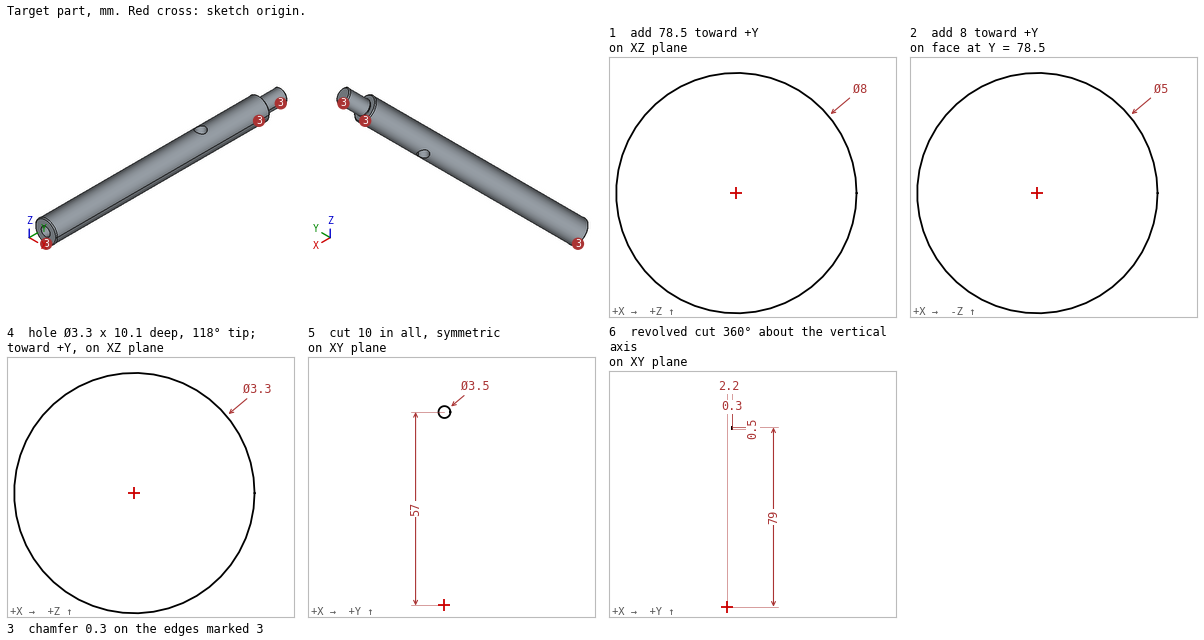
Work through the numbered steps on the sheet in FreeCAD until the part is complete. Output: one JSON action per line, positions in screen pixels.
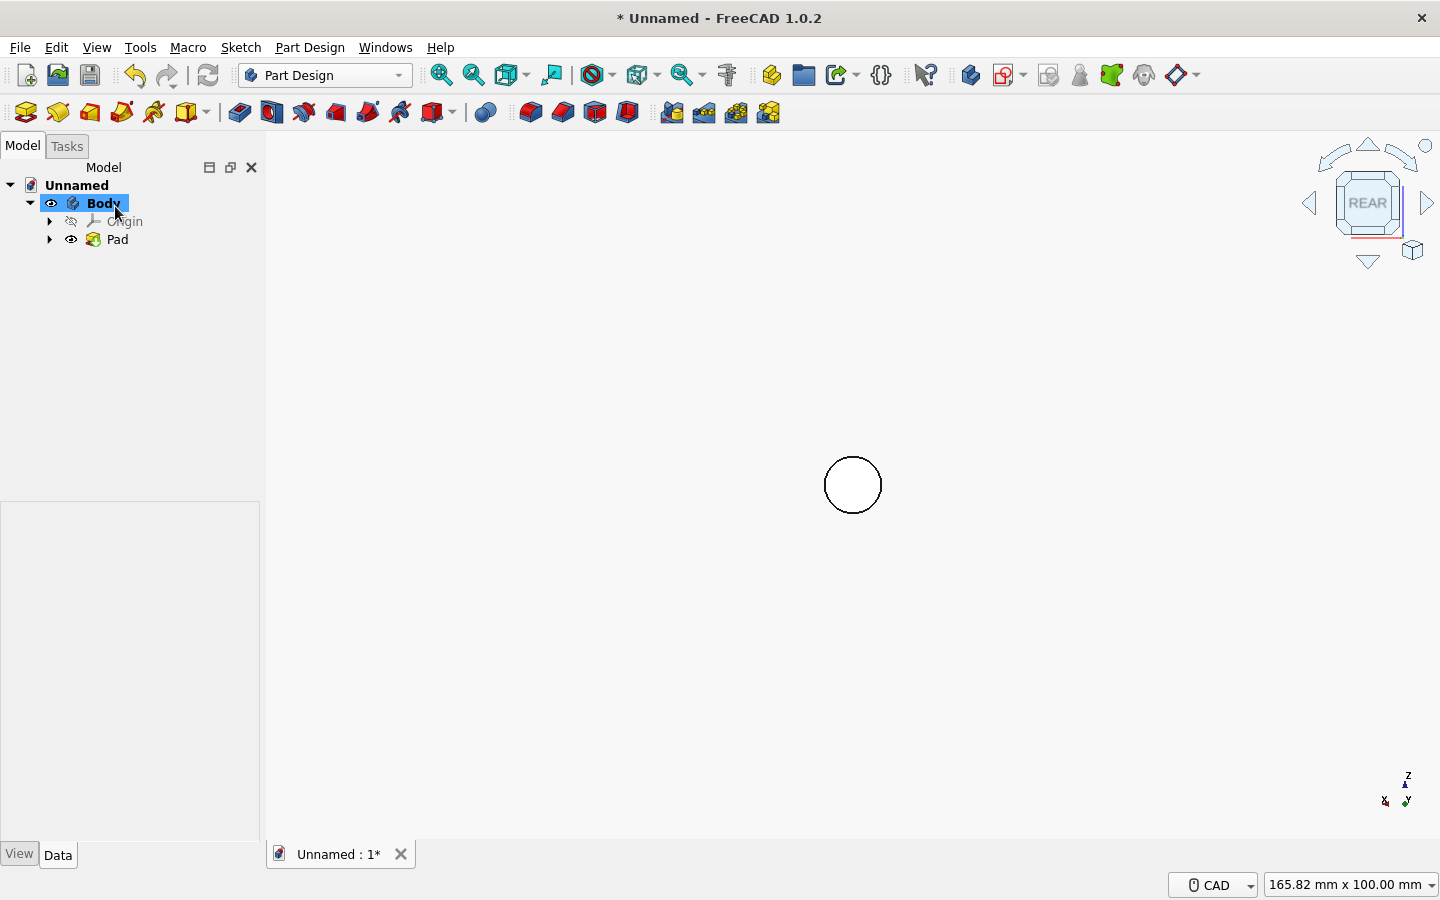
{"action": "left_click", "coordinate": [442, 76]}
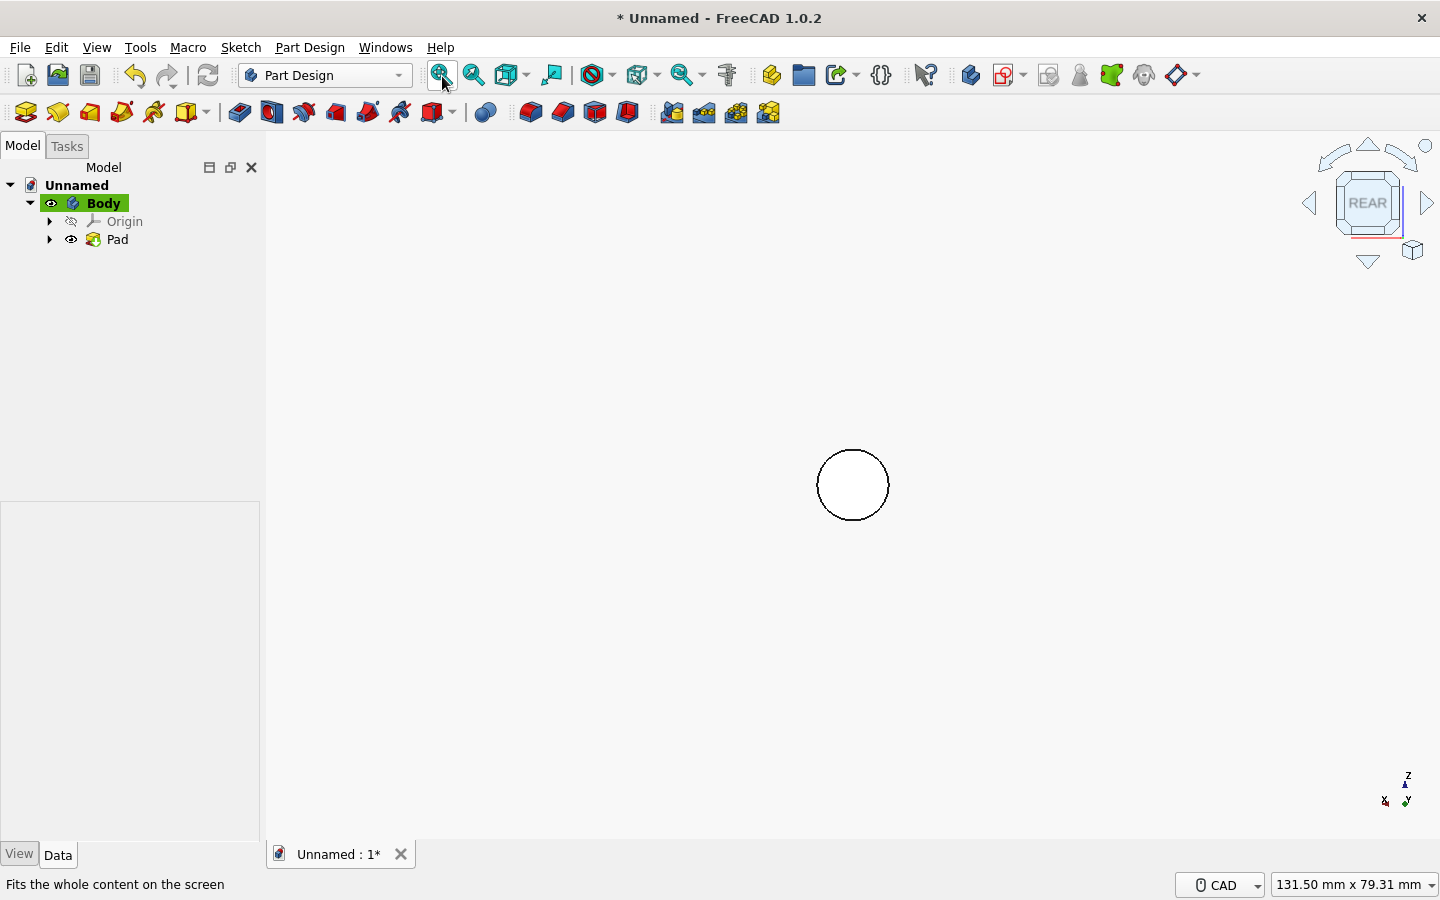
{"action": "left_click", "coordinate": [853, 484]}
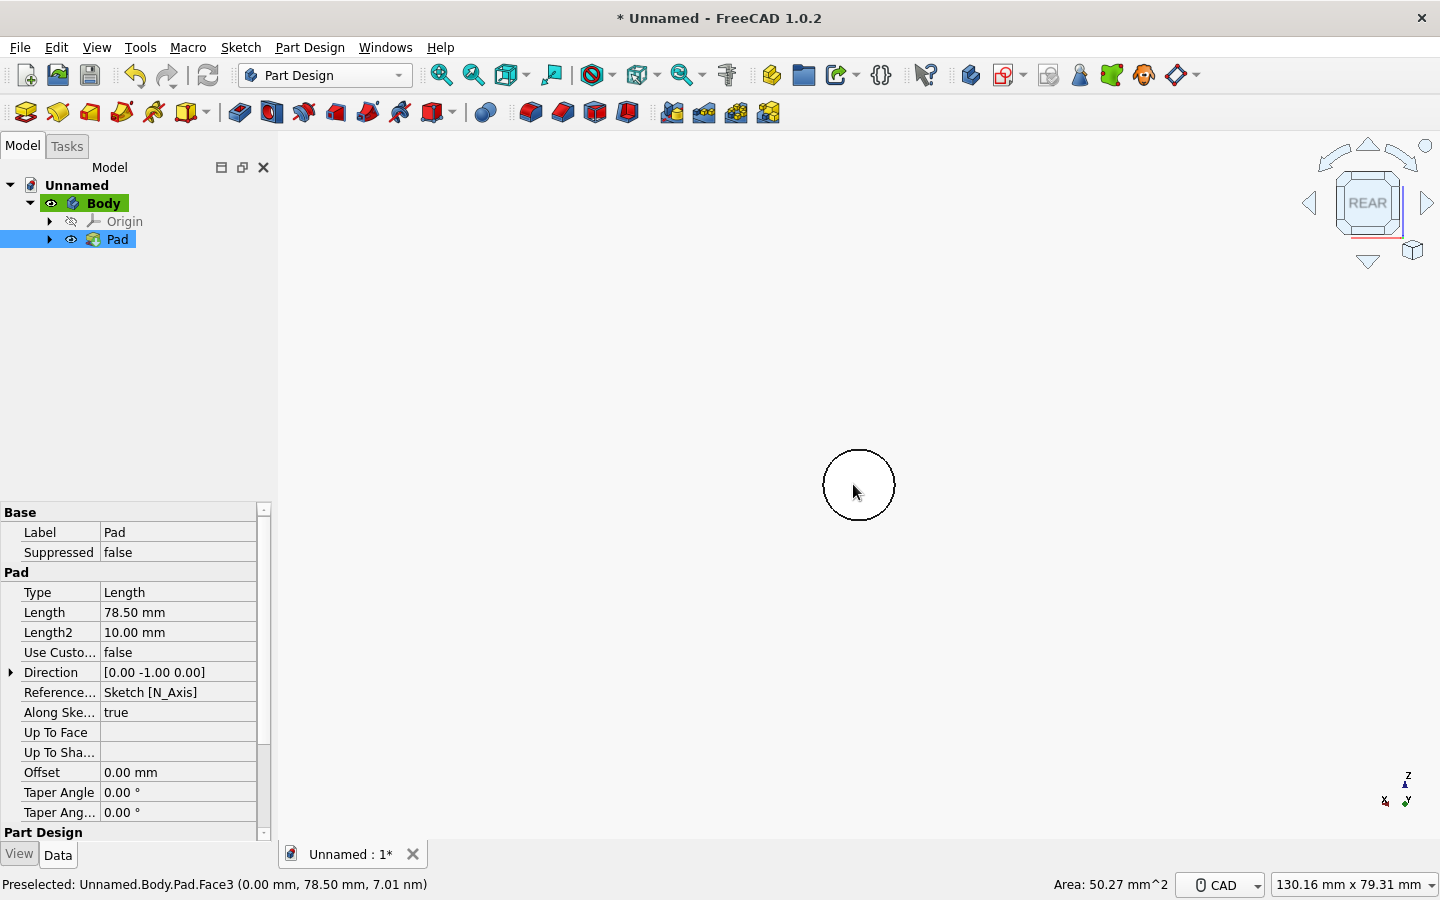
{"action": "left_click", "coordinate": [1004, 76]}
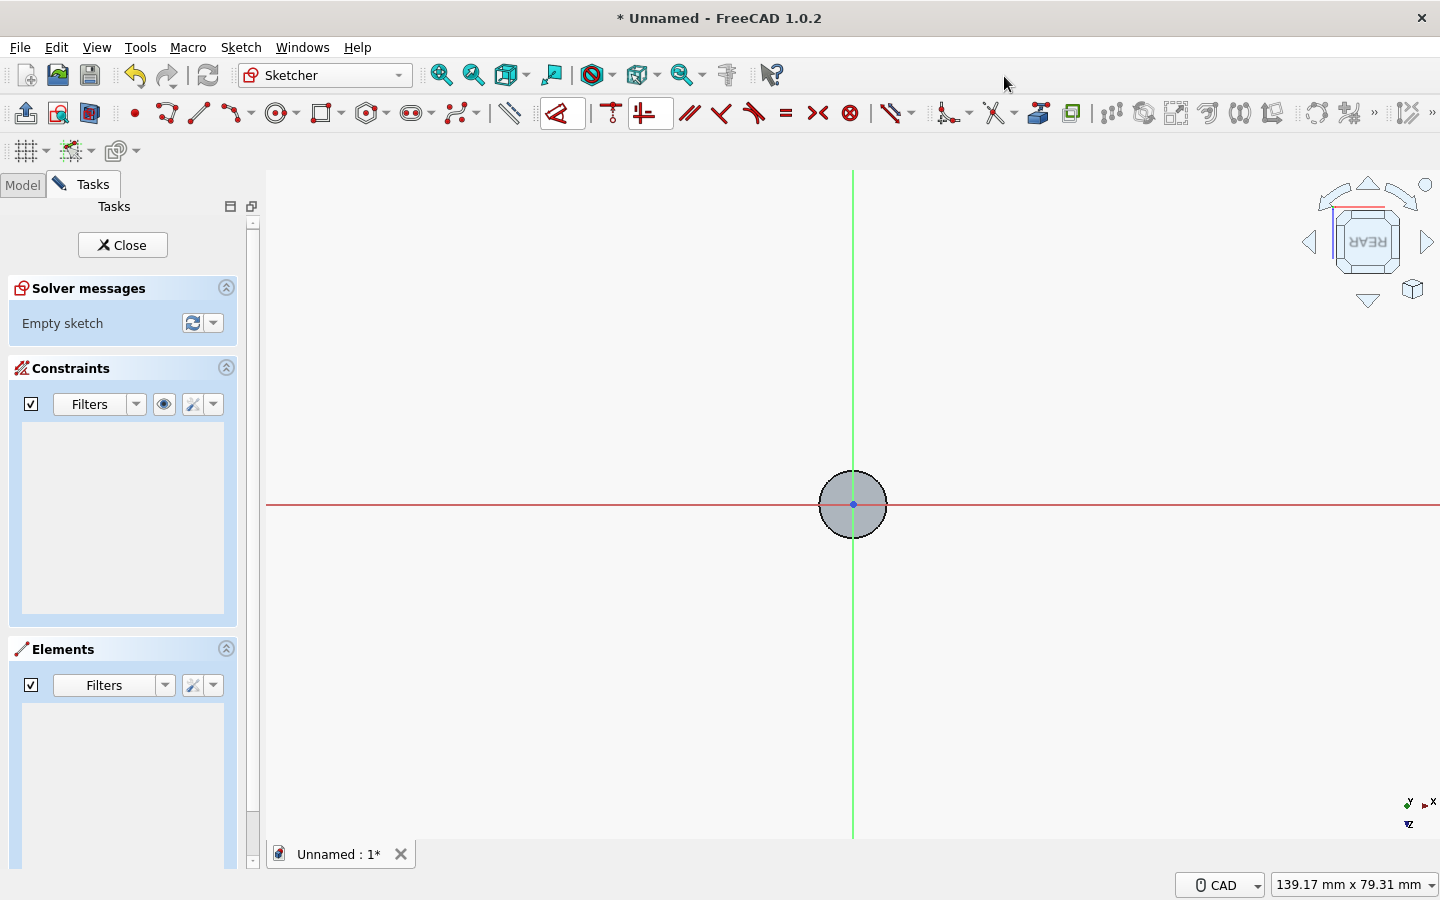
{"action": "scroll", "coordinate": [860, 504], "scroll_direction": "up", "scroll_amount": 12}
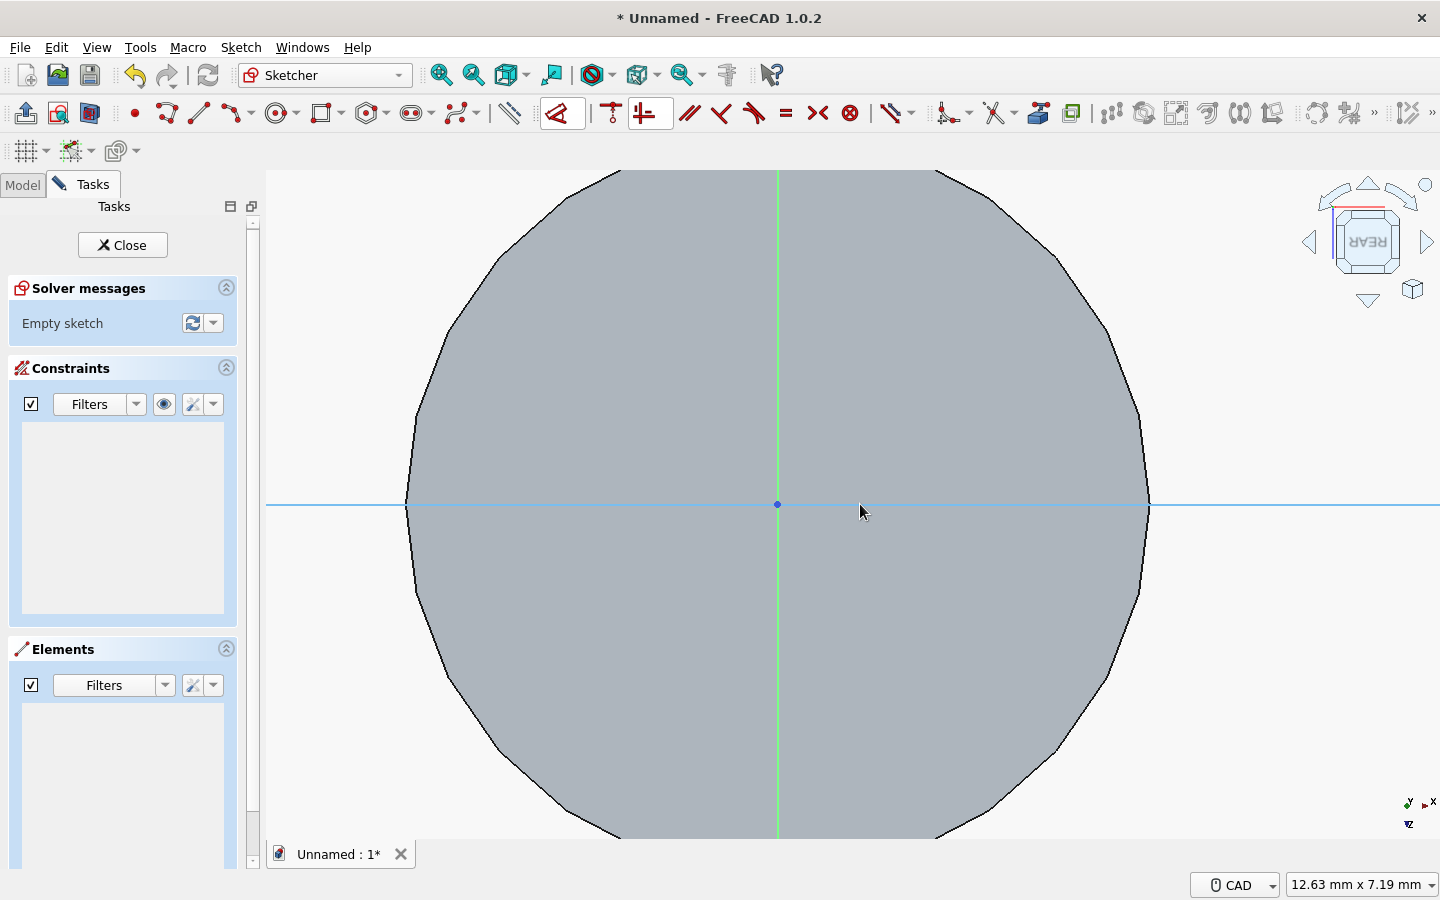
{"action": "key", "text": "g c"}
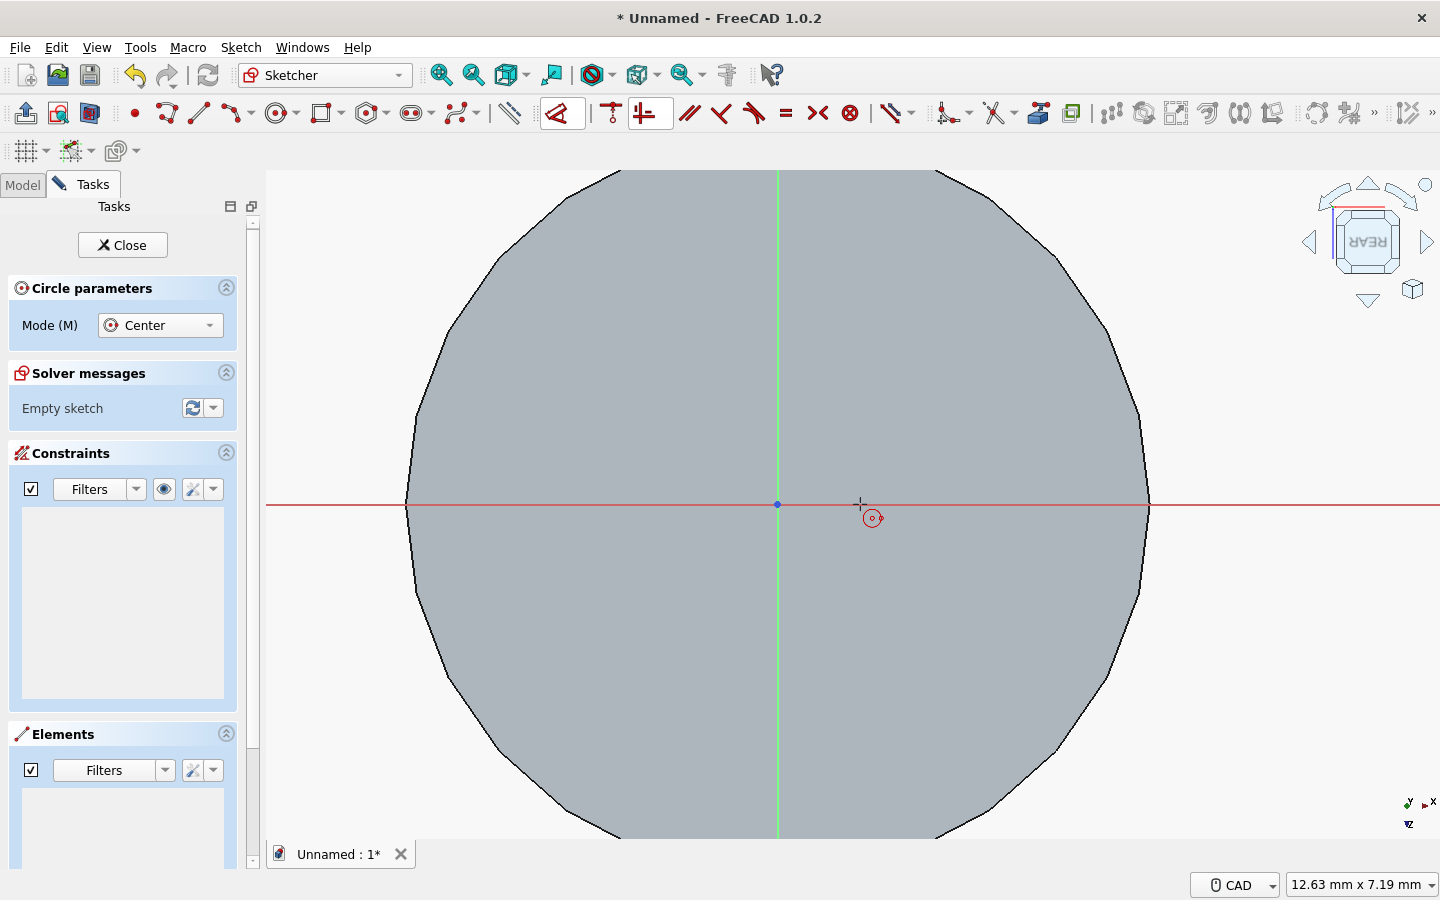
{"action": "left_click", "coordinate": [778, 504]}
{"action": "left_click", "coordinate": [942, 340]}
{"action": "key", "text": "Escape"}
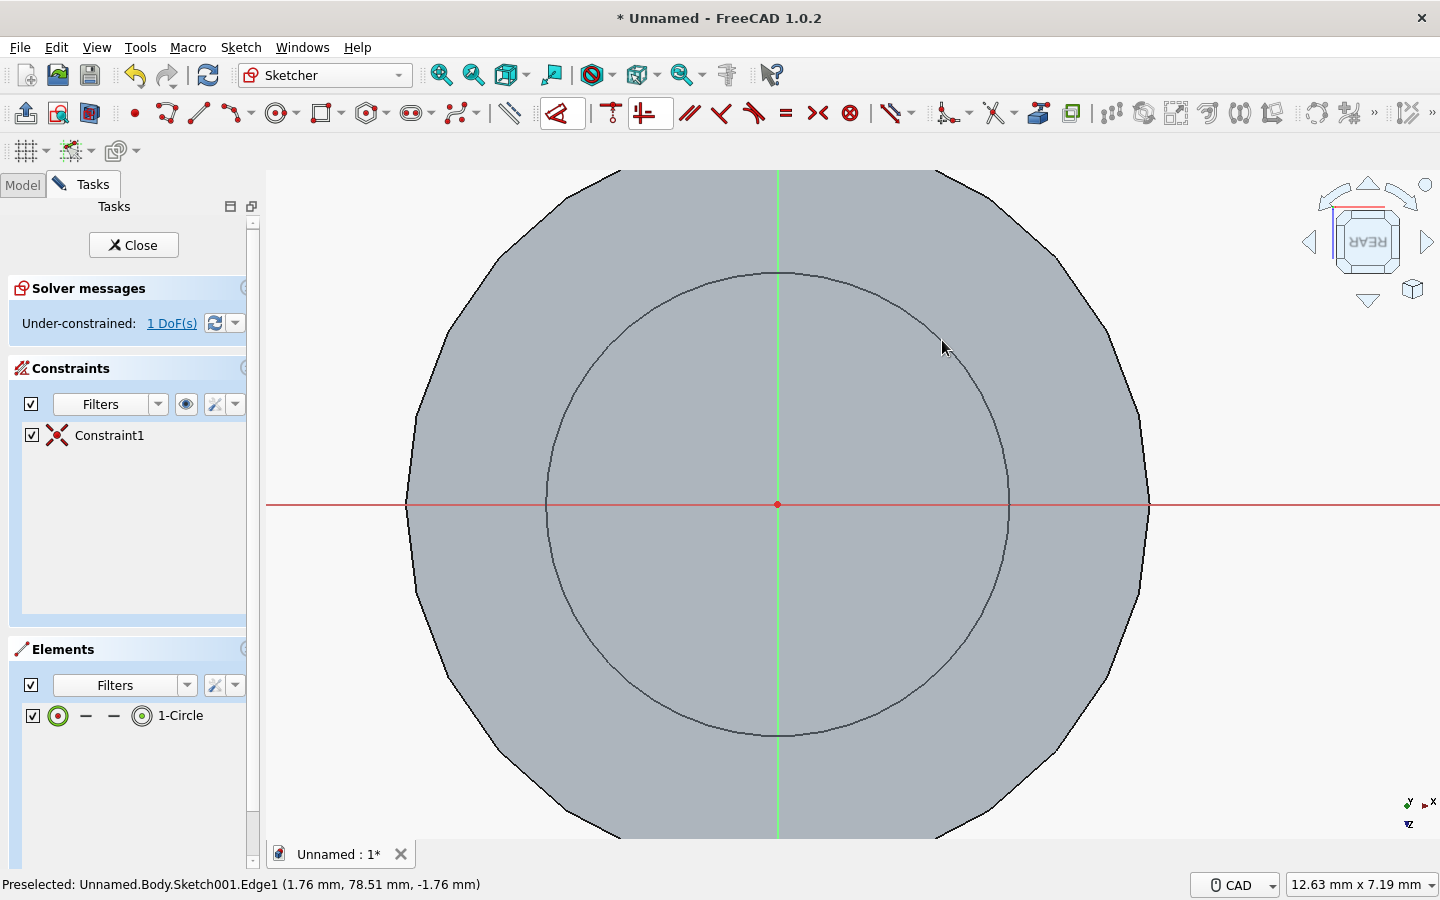
{"action": "left_click", "coordinate": [556, 114]}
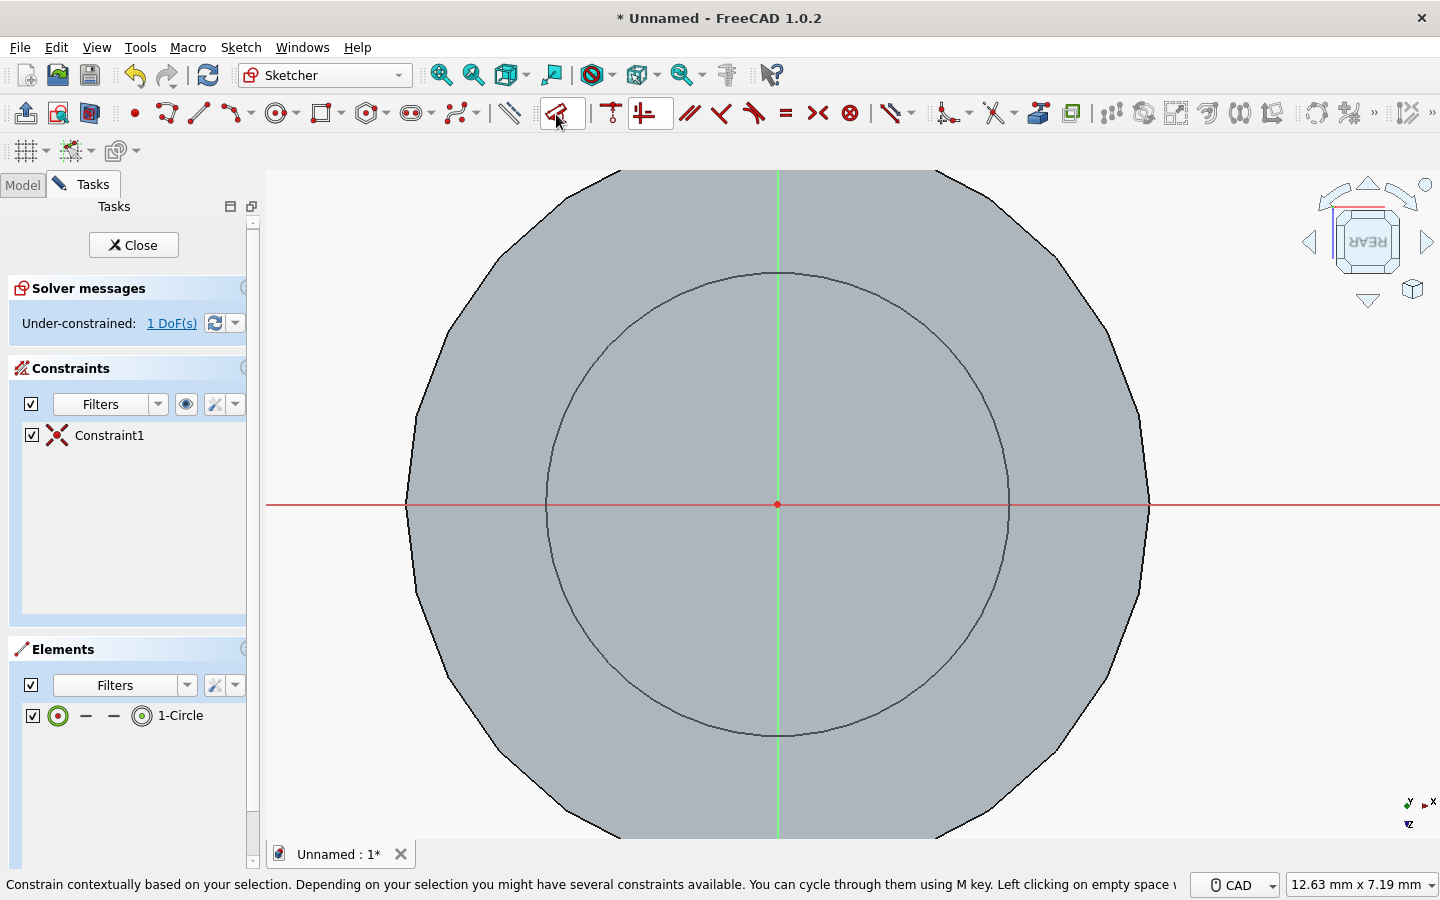
{"action": "left_click", "coordinate": [941, 340]}
{"action": "left_click", "coordinate": [964, 317]}